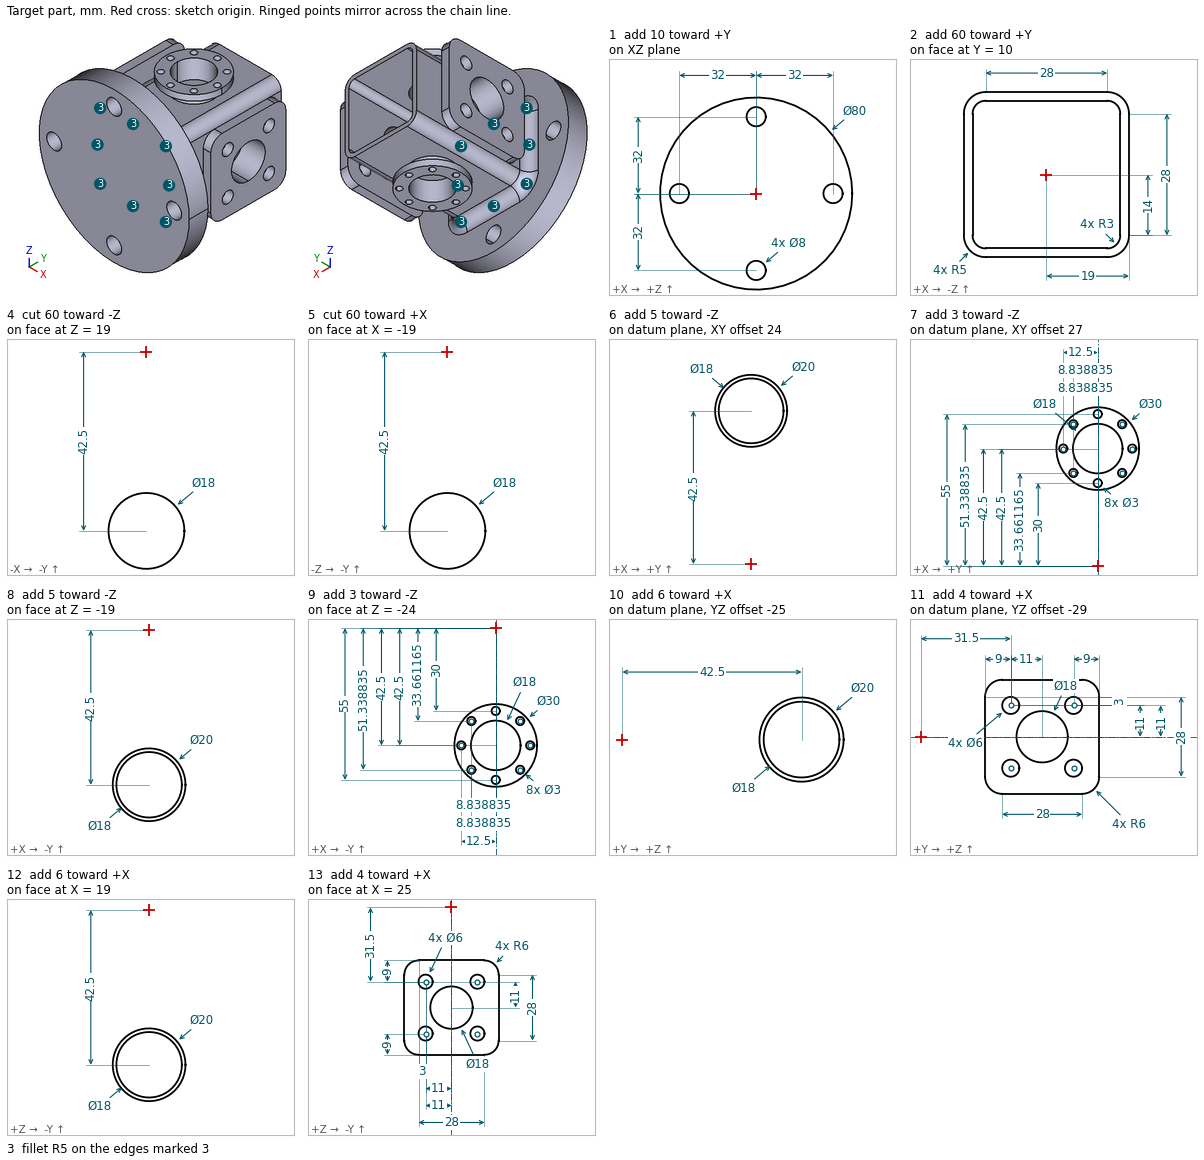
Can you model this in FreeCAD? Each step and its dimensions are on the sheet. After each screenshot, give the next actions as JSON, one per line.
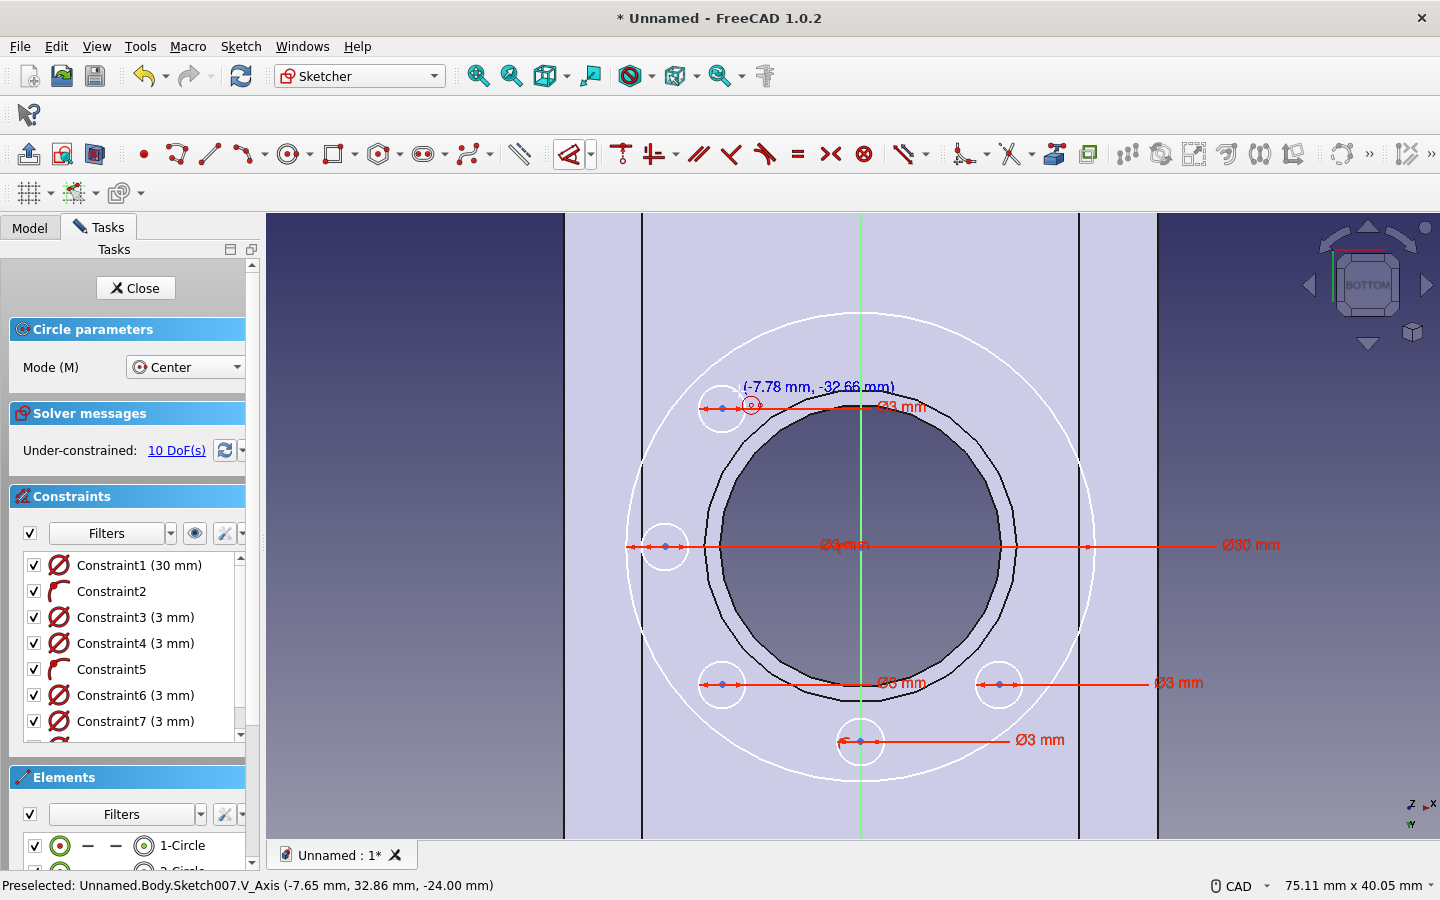
{"action": "left_click", "coordinate": [861, 547]}
{"action": "mouse_move", "coordinate": [960, 446]}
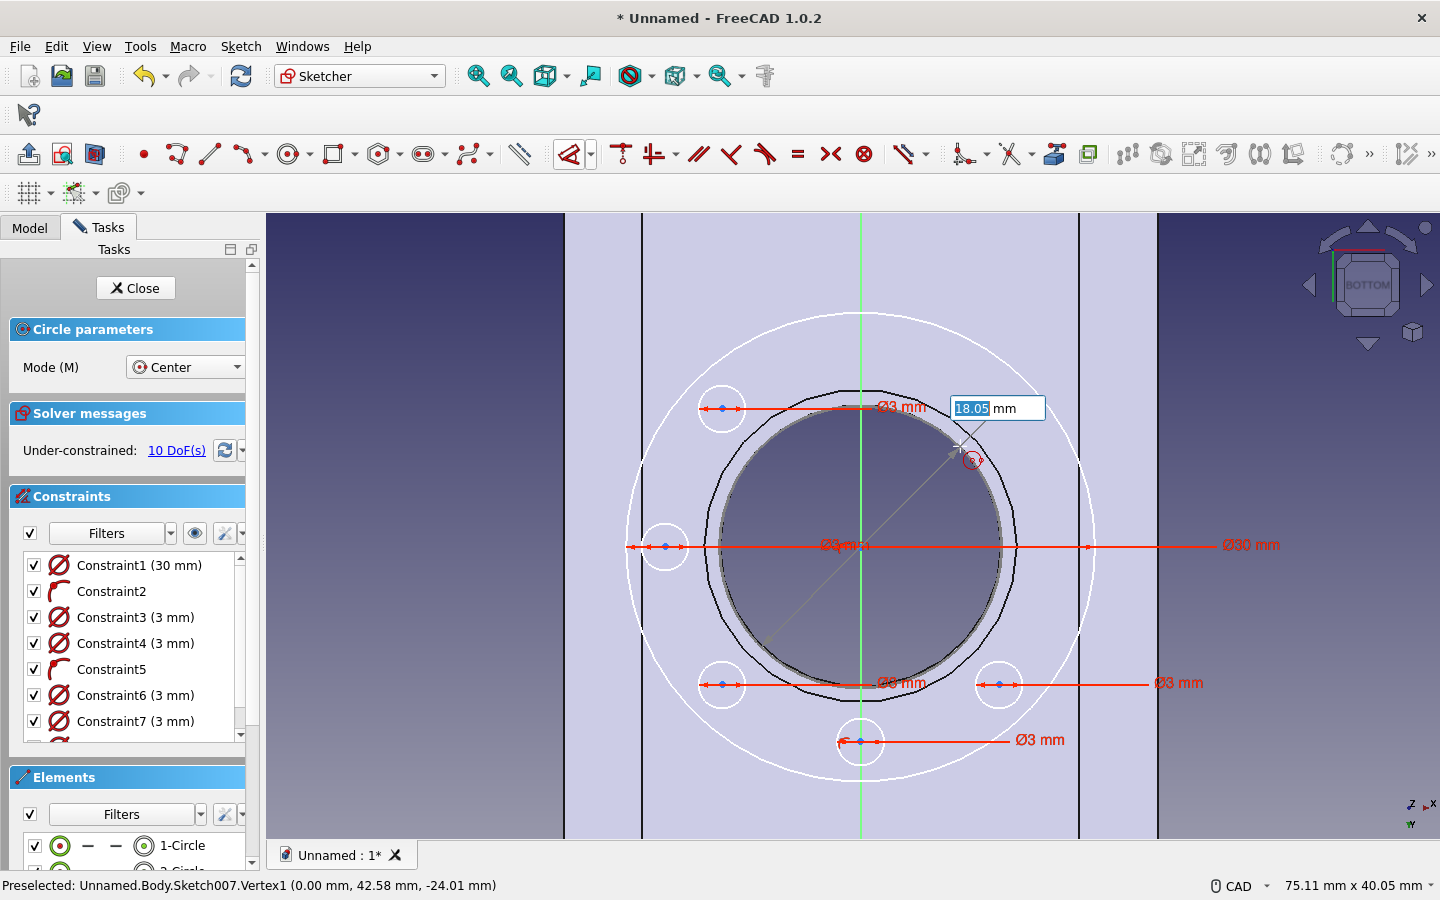
{"action": "type", "text": "18"}
{"action": "key", "text": "Return"}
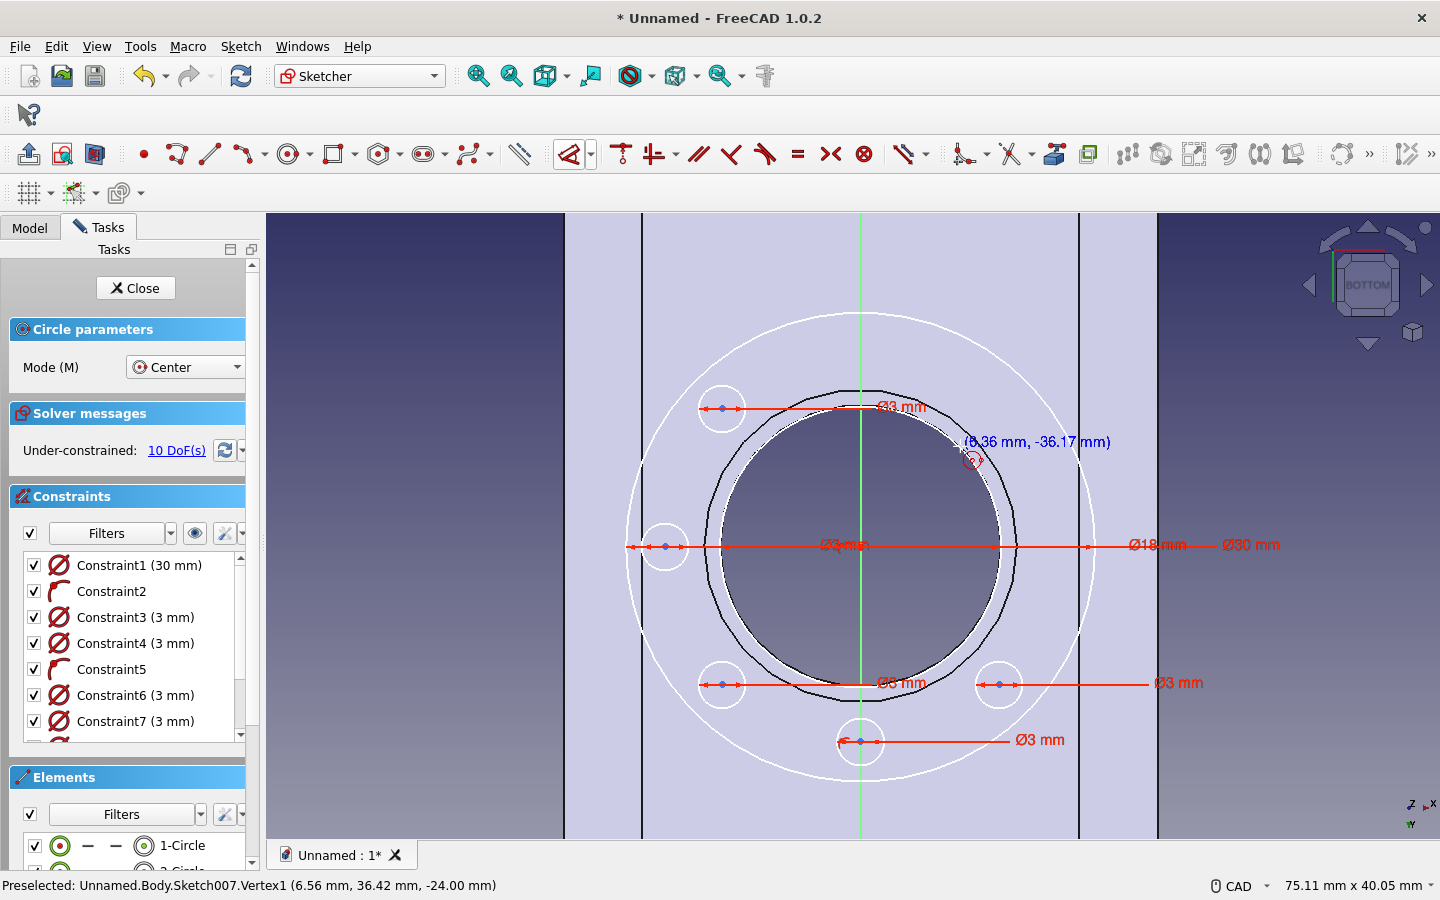
{"action": "left_click", "coordinate": [1056, 546]}
{"action": "mouse_move", "coordinate": [1073, 529]}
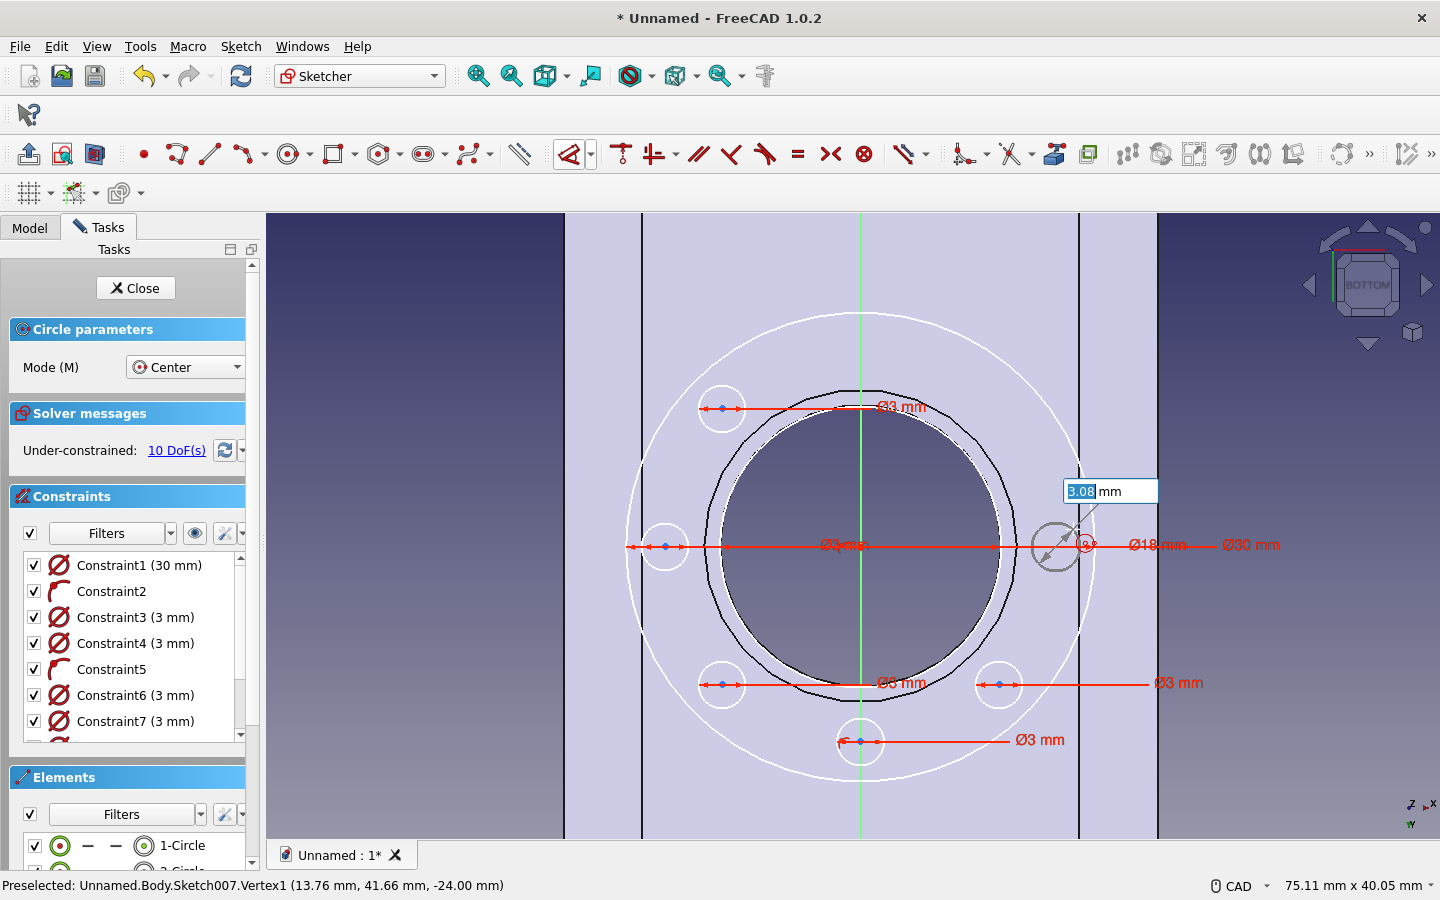
{"action": "type", "text": "3"}
{"action": "key", "text": "Return"}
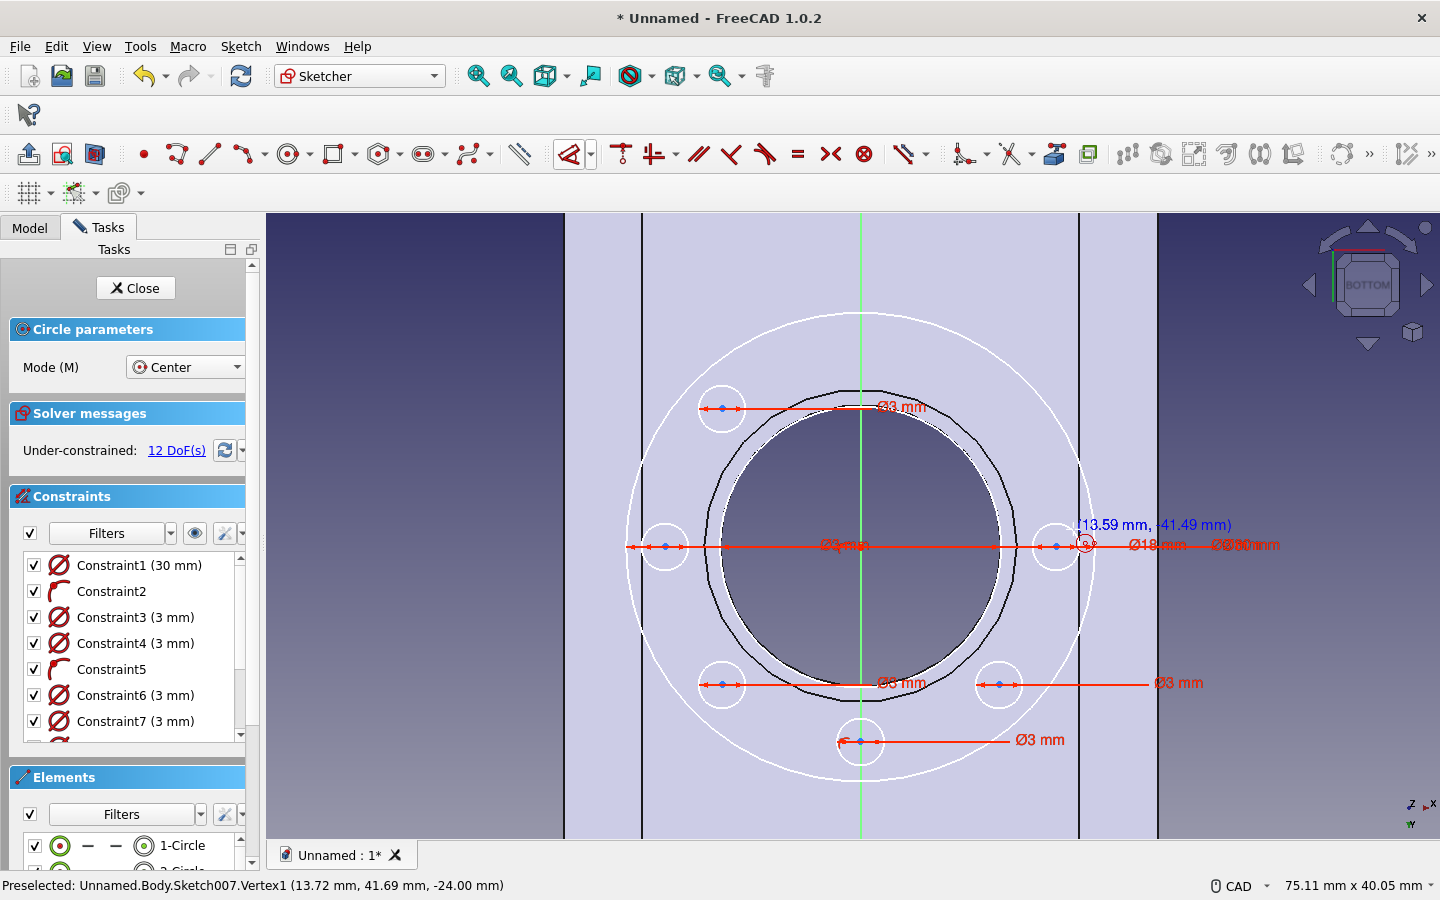
{"action": "left_click", "coordinate": [861, 350]}
{"action": "mouse_move", "coordinate": [877, 334]}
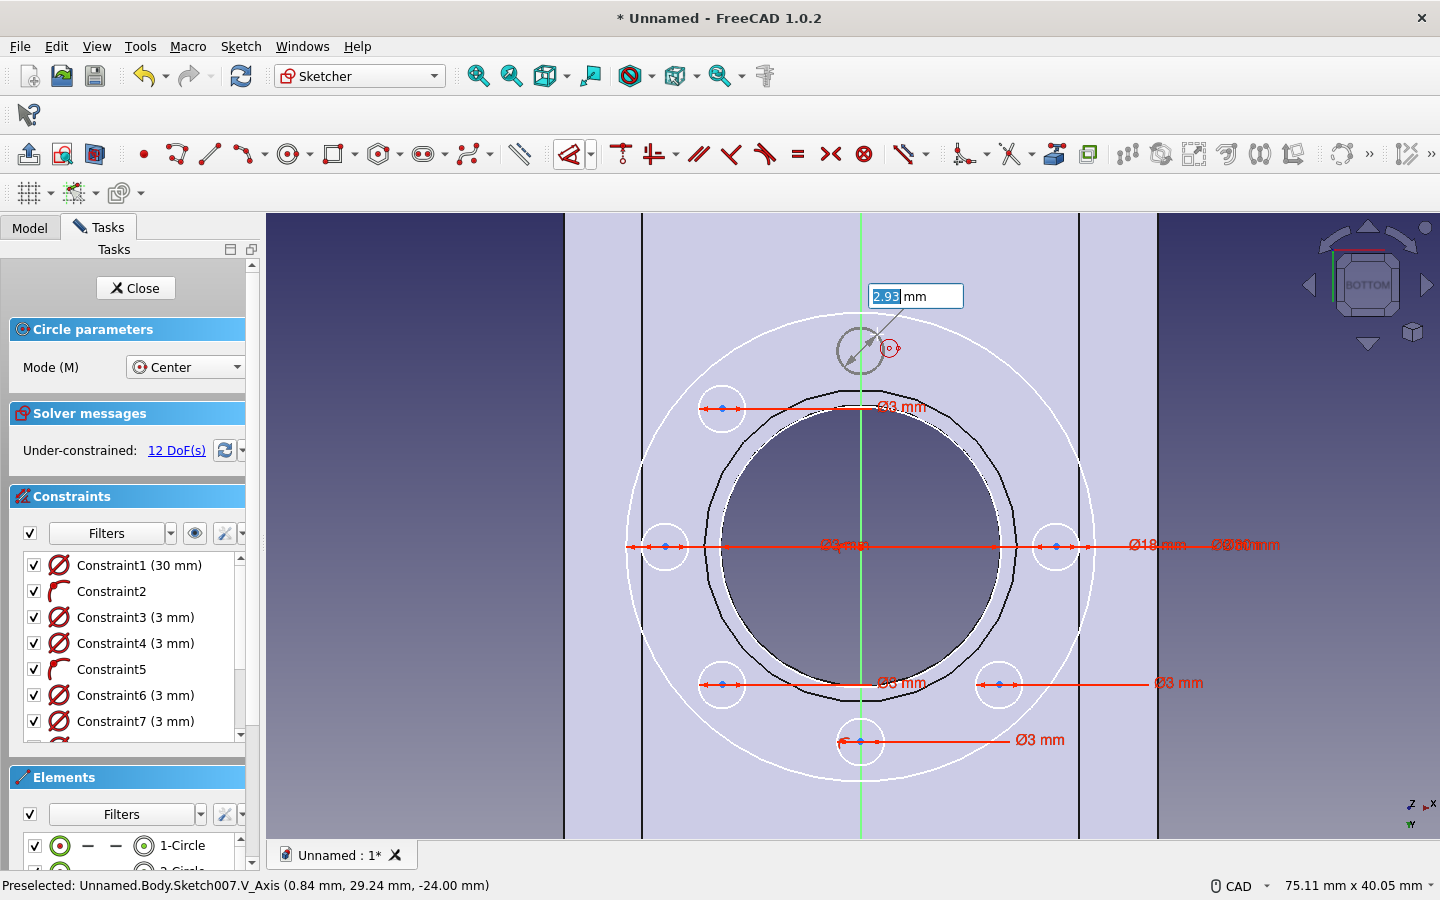
{"action": "type", "text": "3"}
{"action": "key", "text": "Return"}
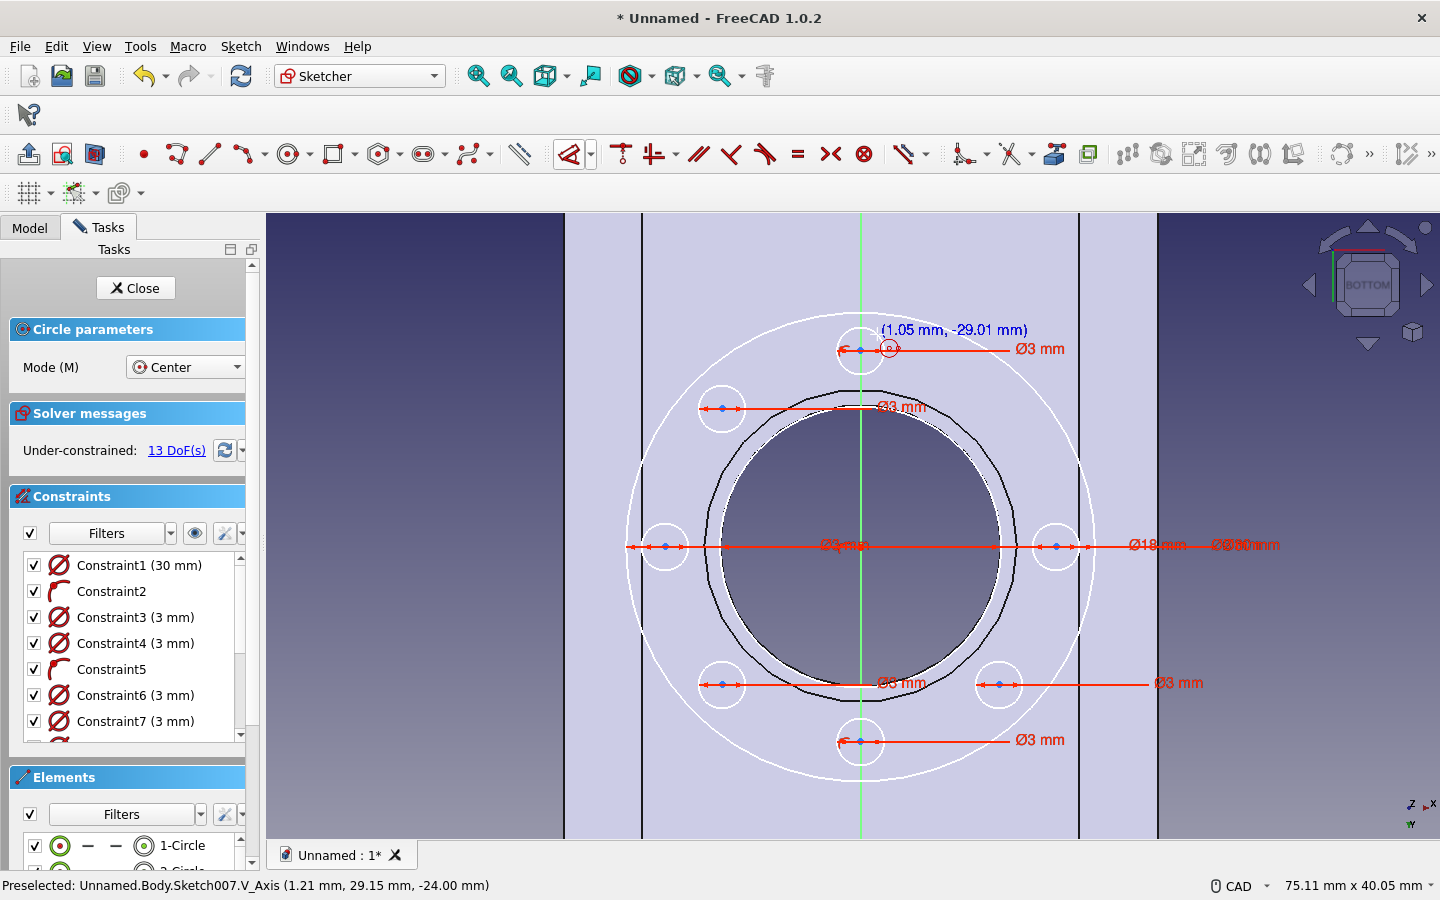
{"action": "left_click", "coordinate": [999, 408]}
{"action": "mouse_move", "coordinate": [1015, 391]}